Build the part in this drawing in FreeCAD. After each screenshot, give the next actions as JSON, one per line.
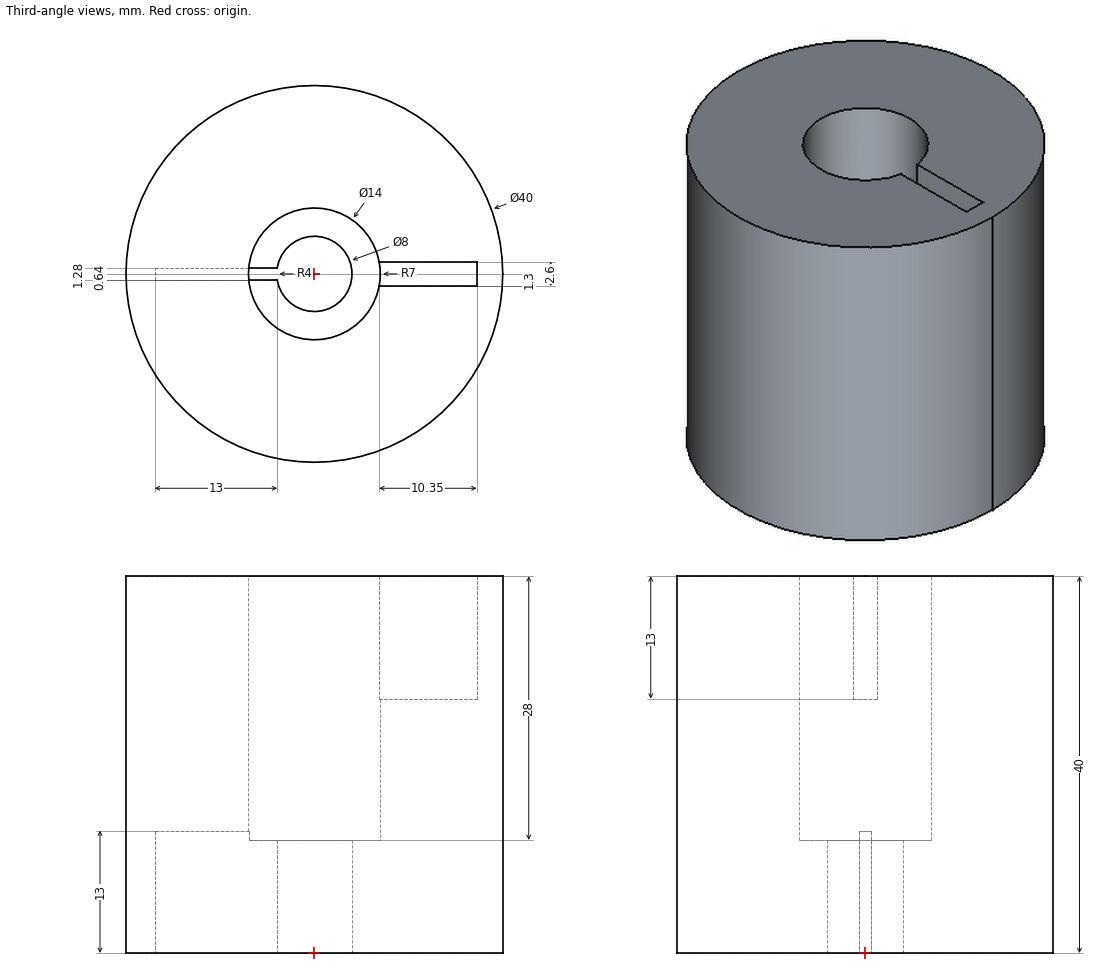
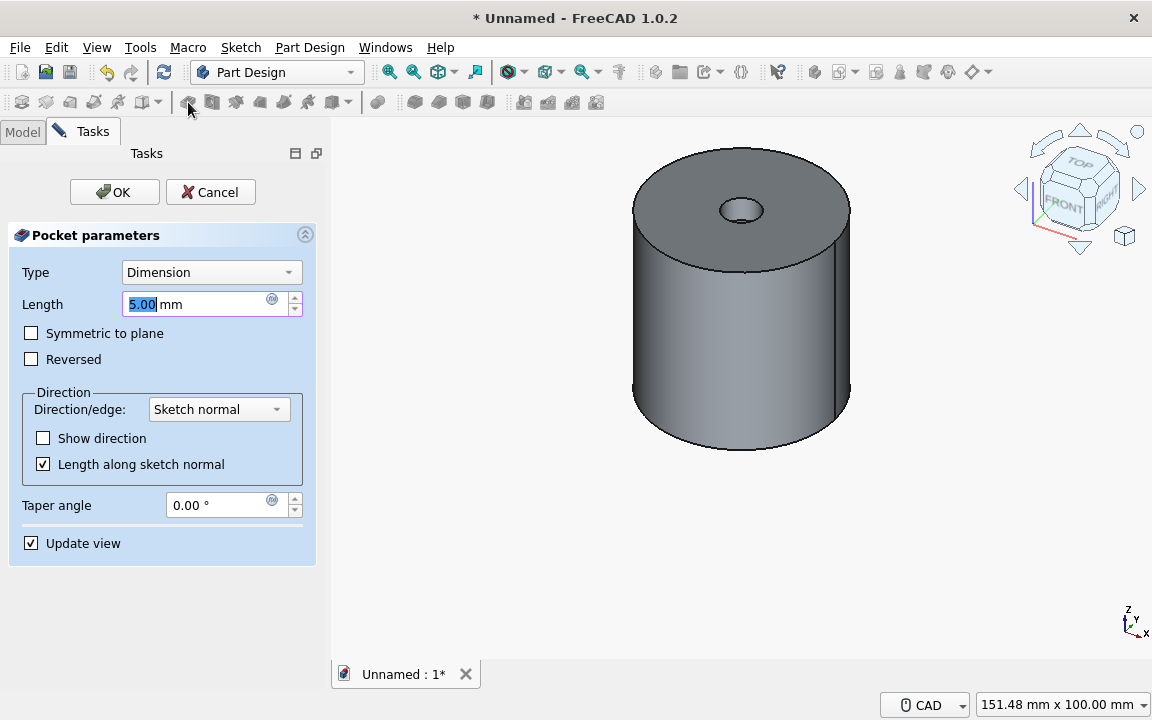
{"action": "left_click", "coordinate": [212, 272]}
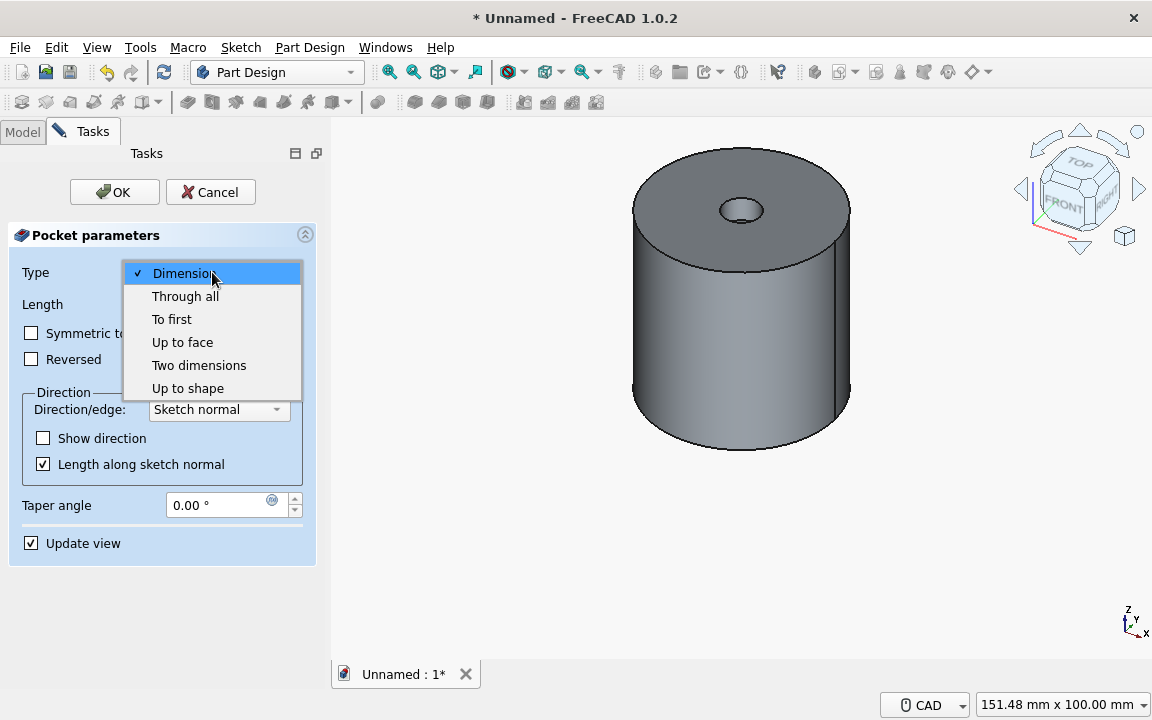
{"action": "left_click", "coordinate": [212, 296]}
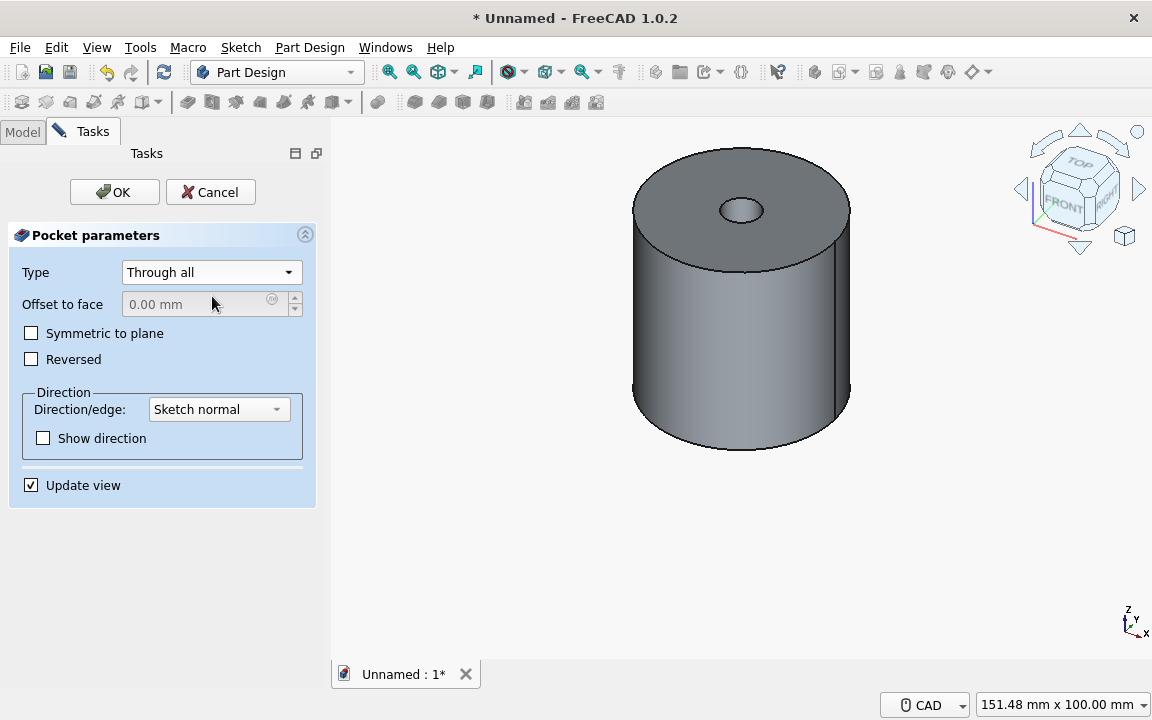
{"action": "left_click", "coordinate": [115, 192]}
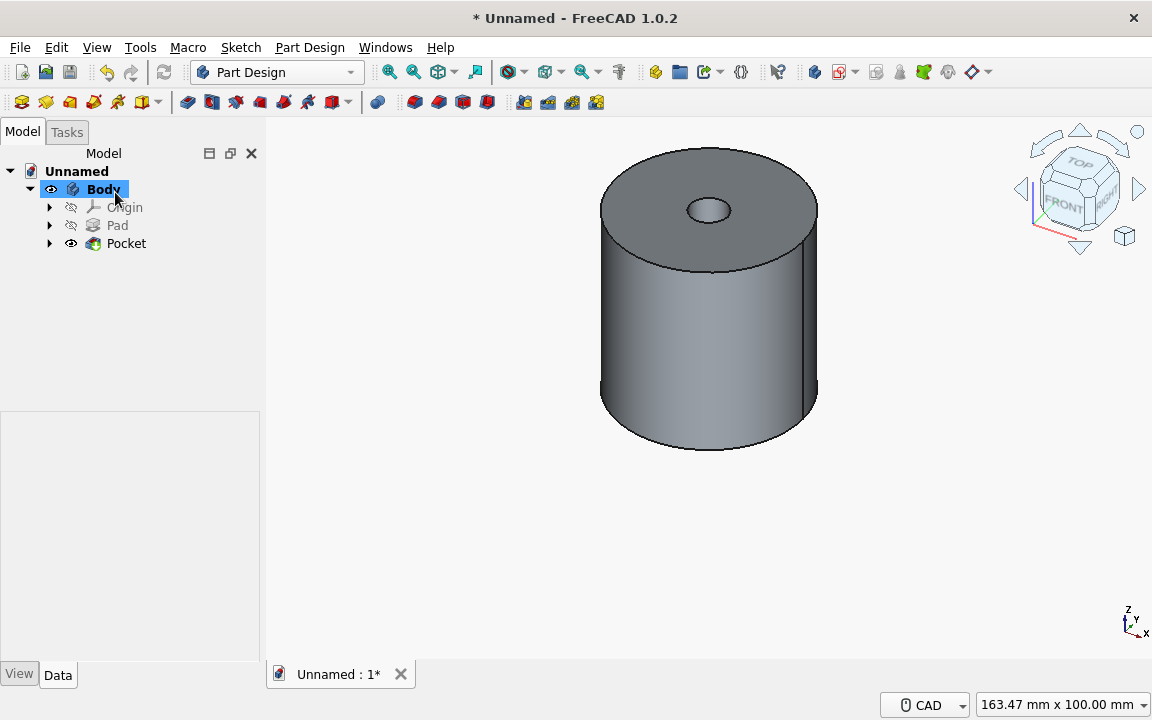
{"action": "left_click", "coordinate": [655, 192]}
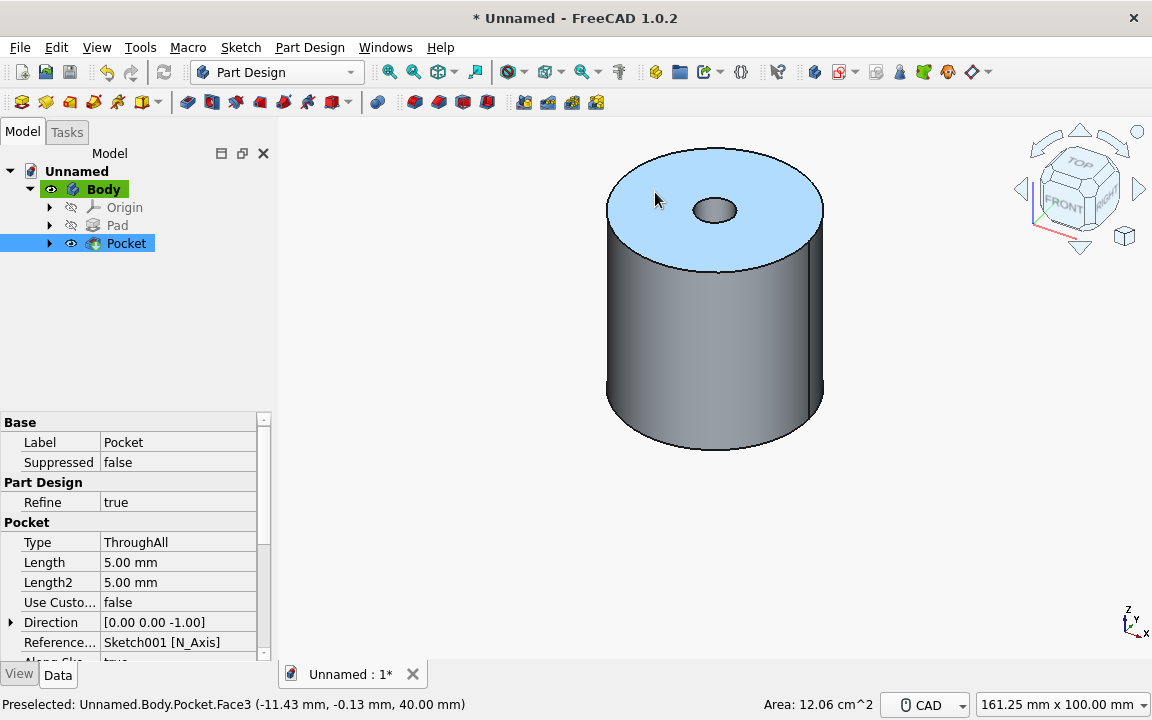
{"action": "left_click", "coordinate": [840, 72]}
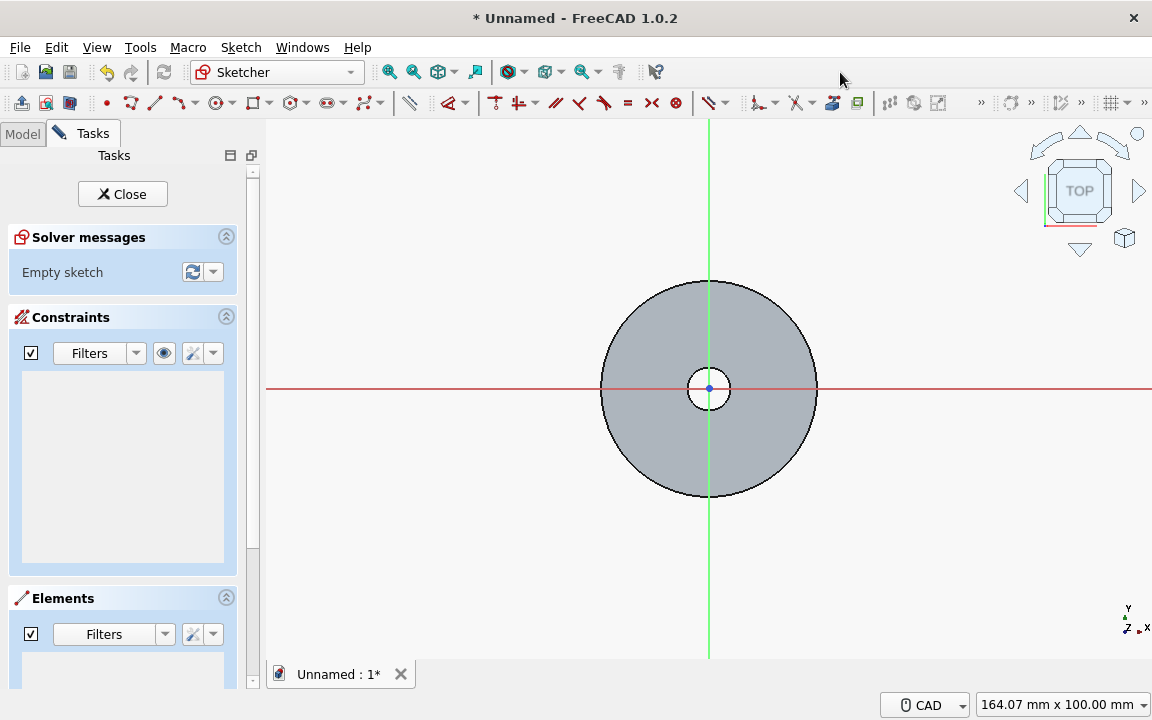
{"action": "scroll", "coordinate": [726, 389], "scroll_direction": "up", "scroll_amount": 8}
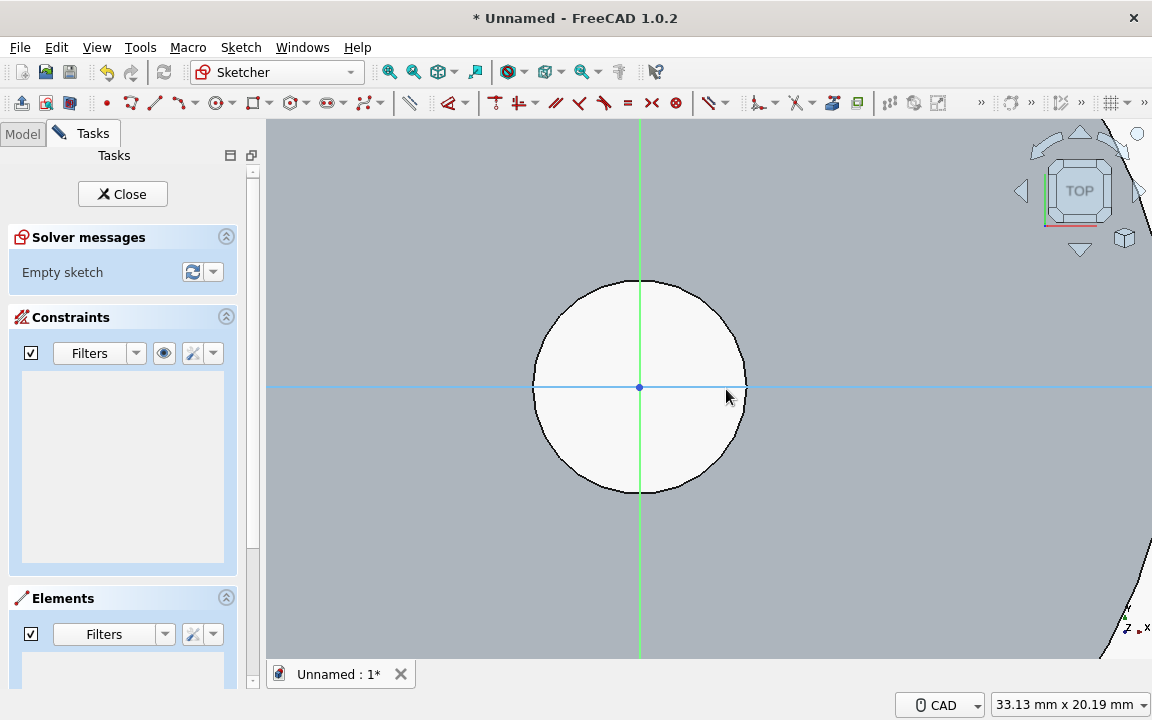
{"action": "key", "text": "g c"}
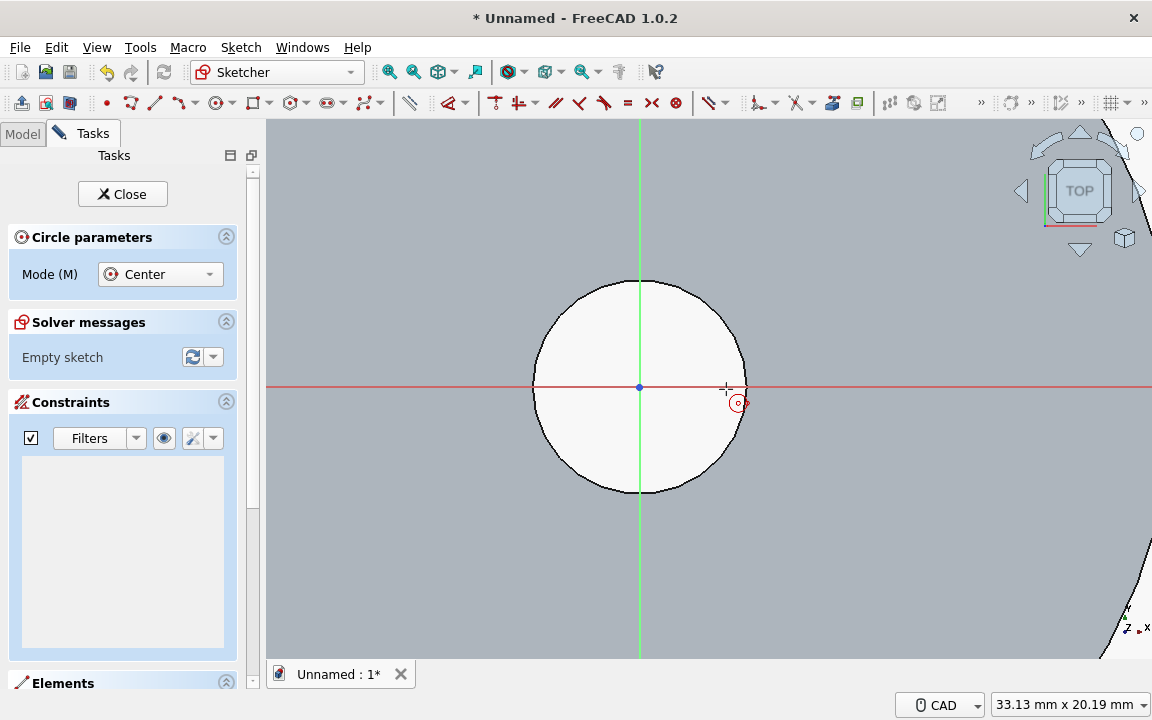
{"action": "left_click", "coordinate": [640, 387]}
{"action": "left_click", "coordinate": [772, 255]}
{"action": "key", "text": "Escape"}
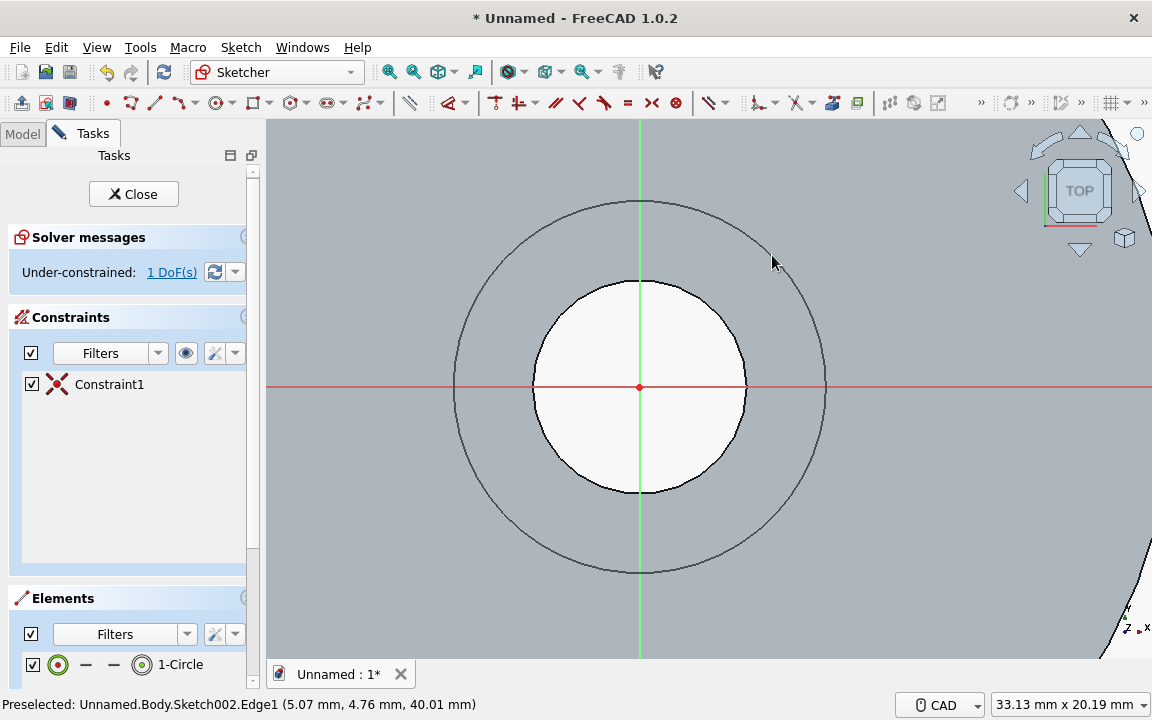
{"action": "key", "text": "d"}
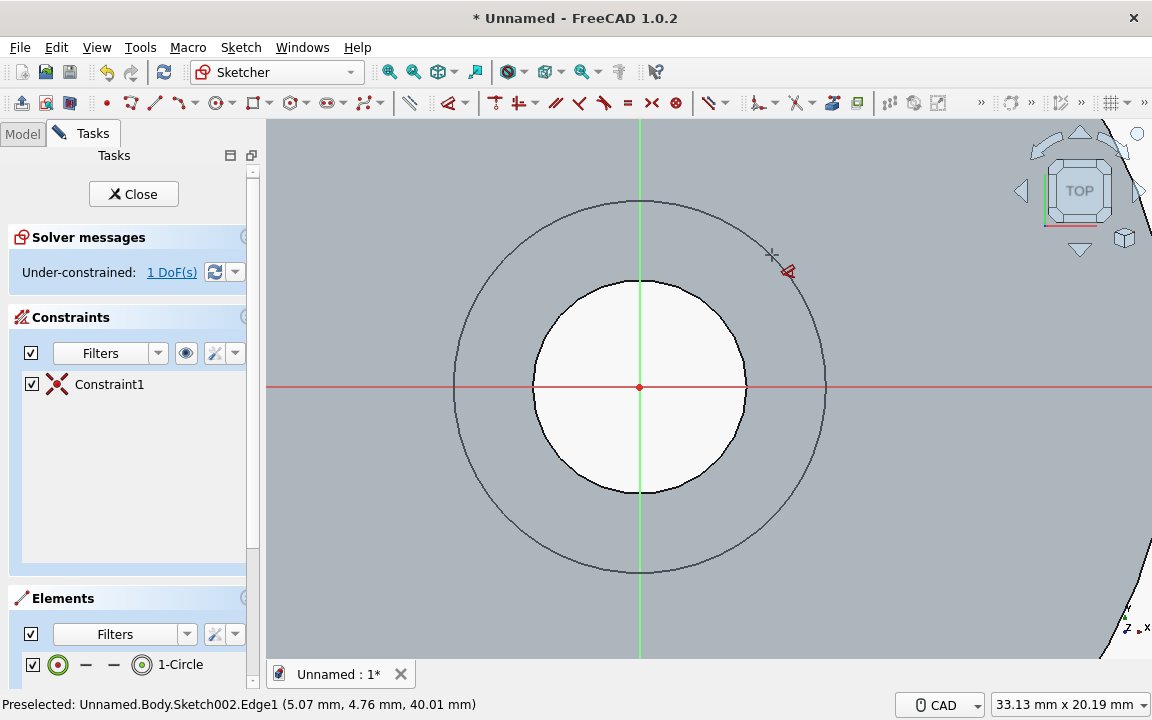
{"action": "left_click", "coordinate": [771, 255]}
{"action": "left_click", "coordinate": [794, 232]}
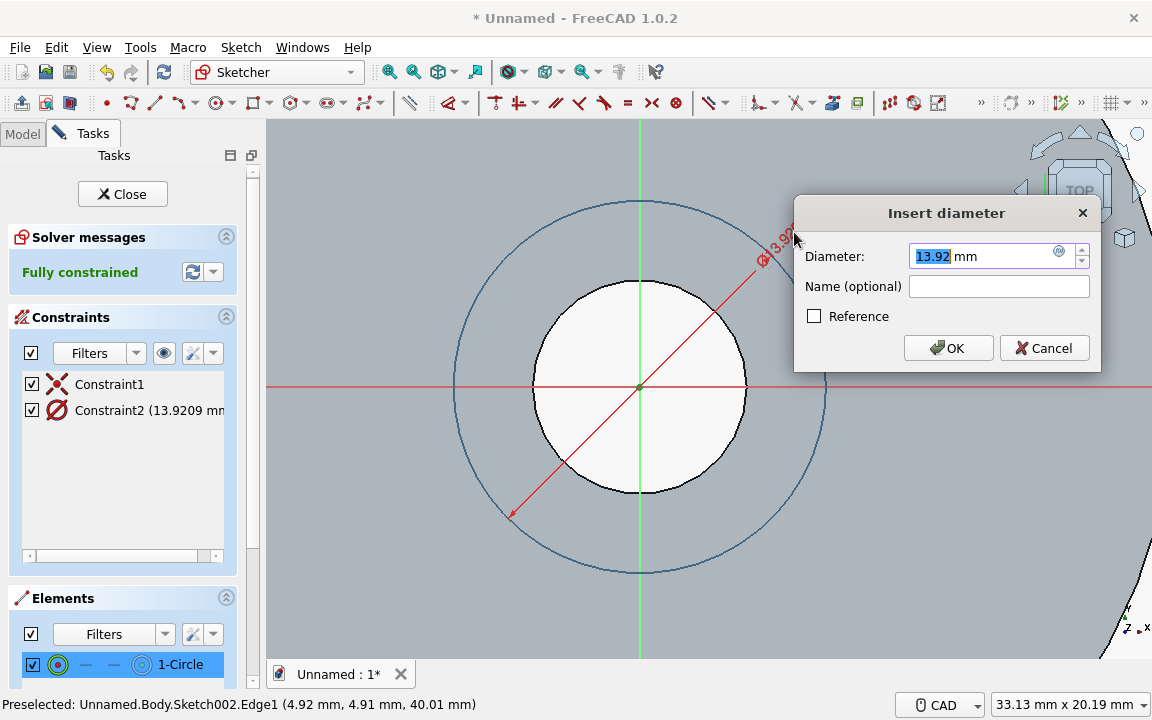
{"action": "type", "text": "14"}
{"action": "key", "text": "Return"}
{"action": "key", "text": "Escape"}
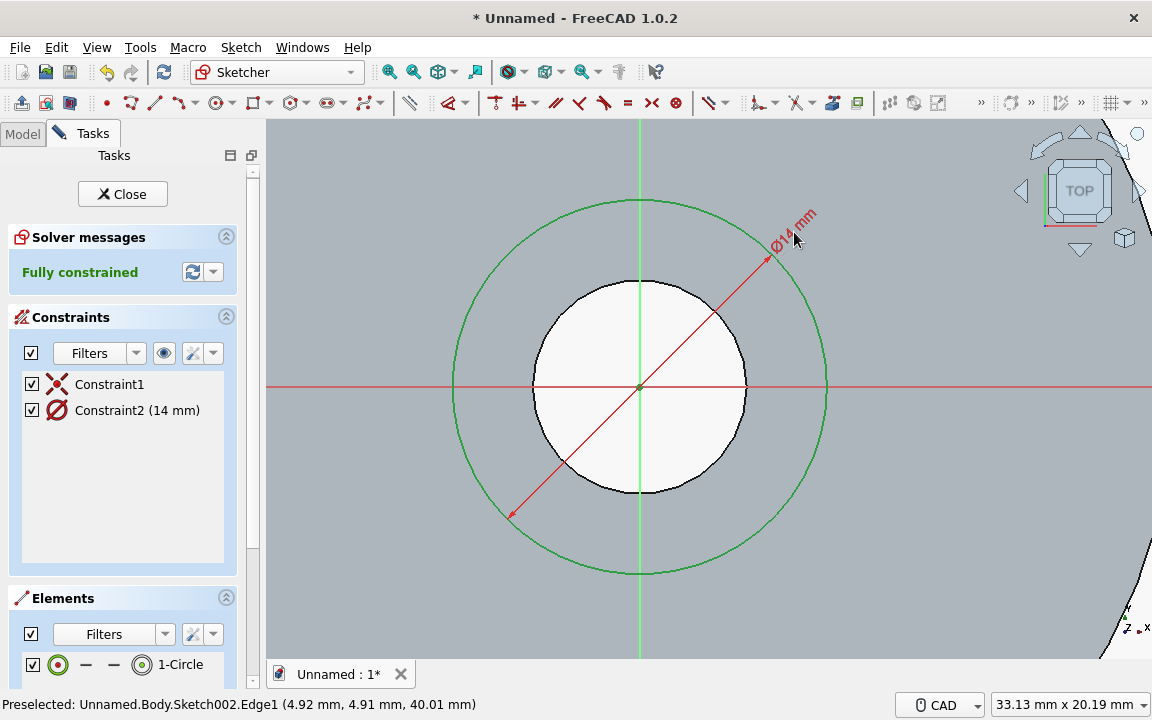
{"action": "left_click", "coordinate": [123, 194]}